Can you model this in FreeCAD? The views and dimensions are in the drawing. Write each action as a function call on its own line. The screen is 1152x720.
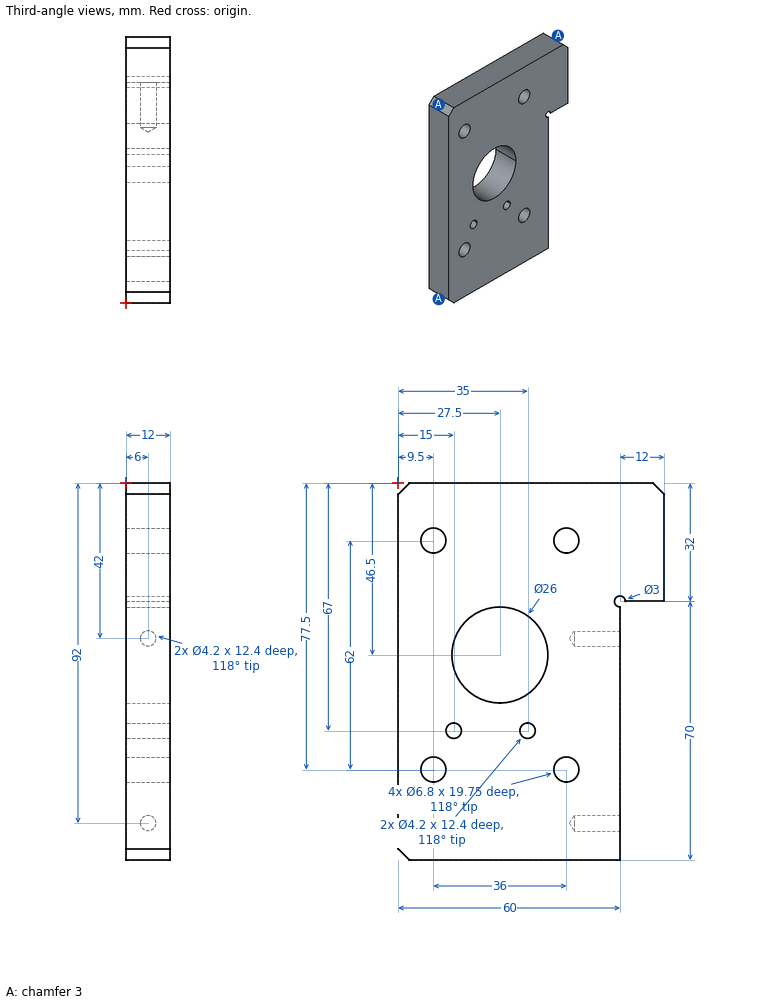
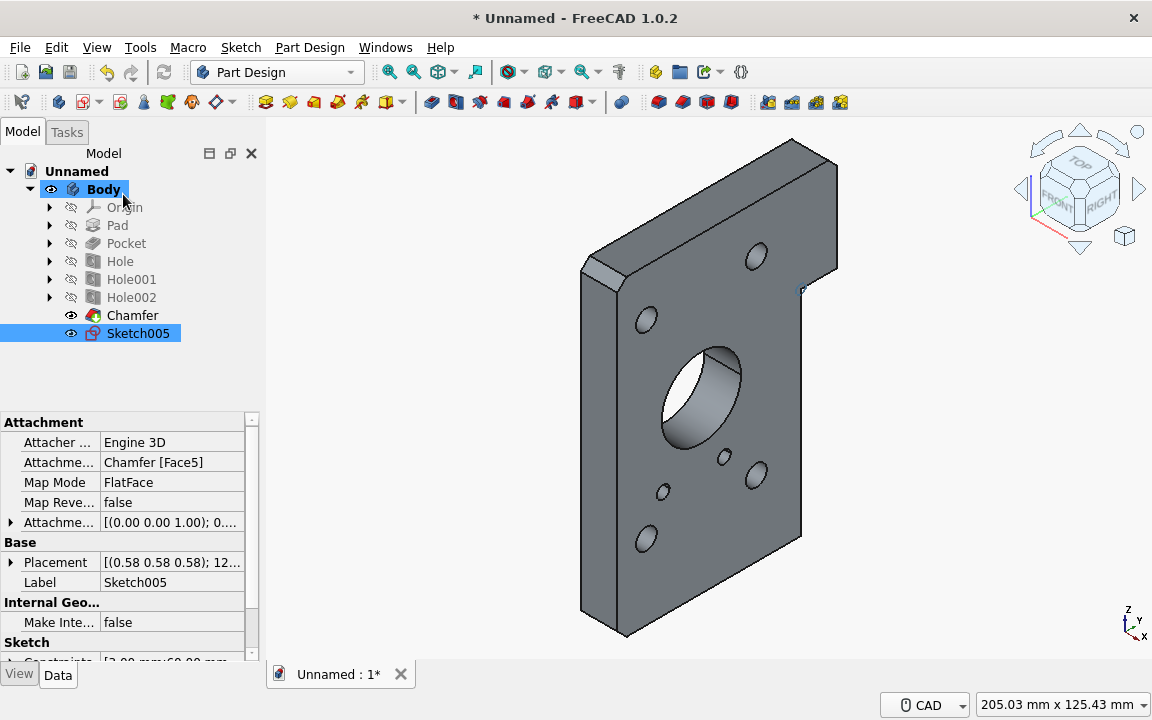
click(432, 102)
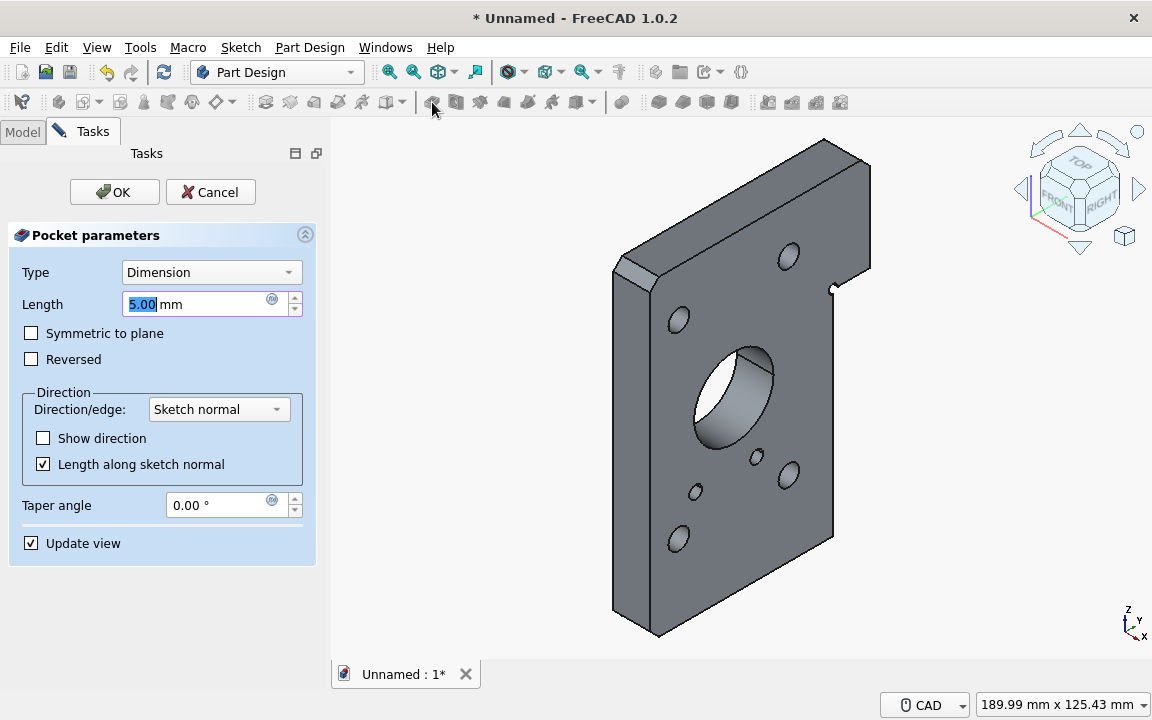
click(212, 272)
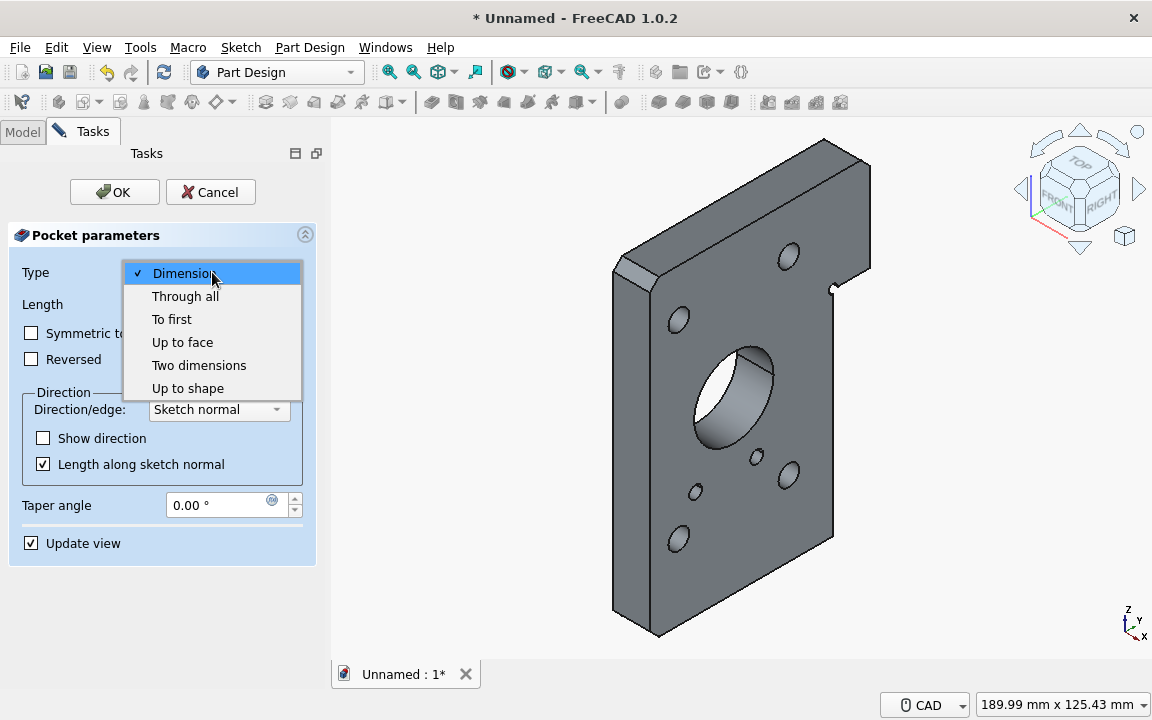
click(212, 296)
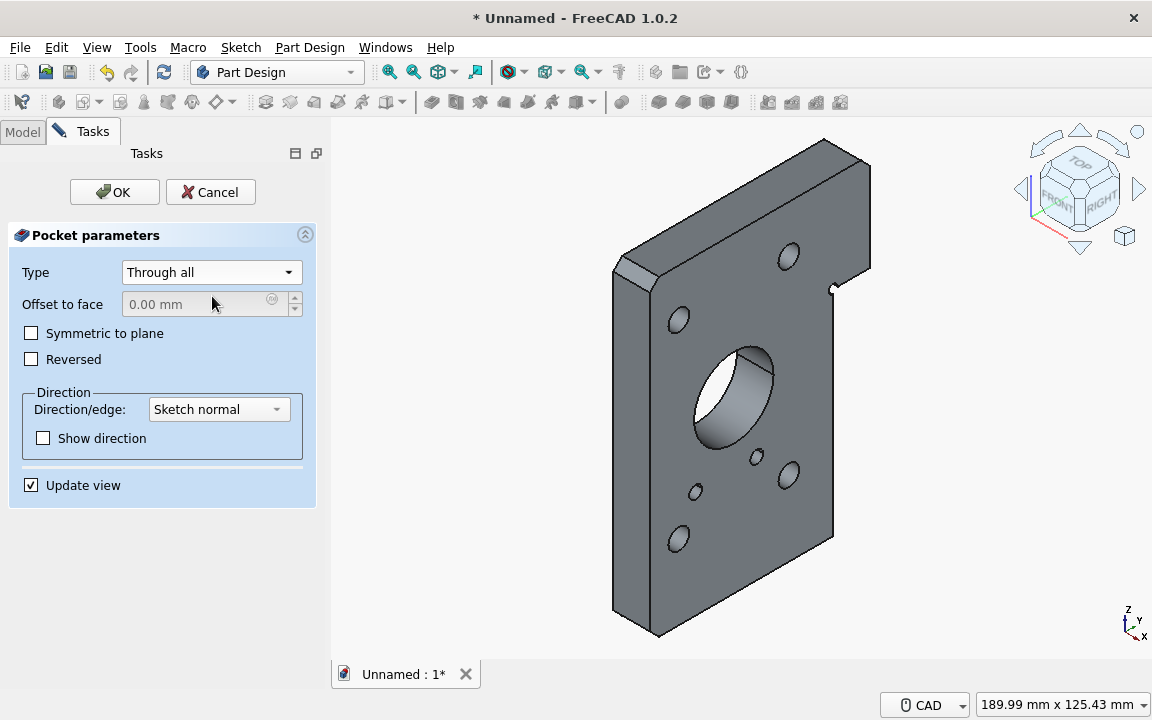
click(115, 192)